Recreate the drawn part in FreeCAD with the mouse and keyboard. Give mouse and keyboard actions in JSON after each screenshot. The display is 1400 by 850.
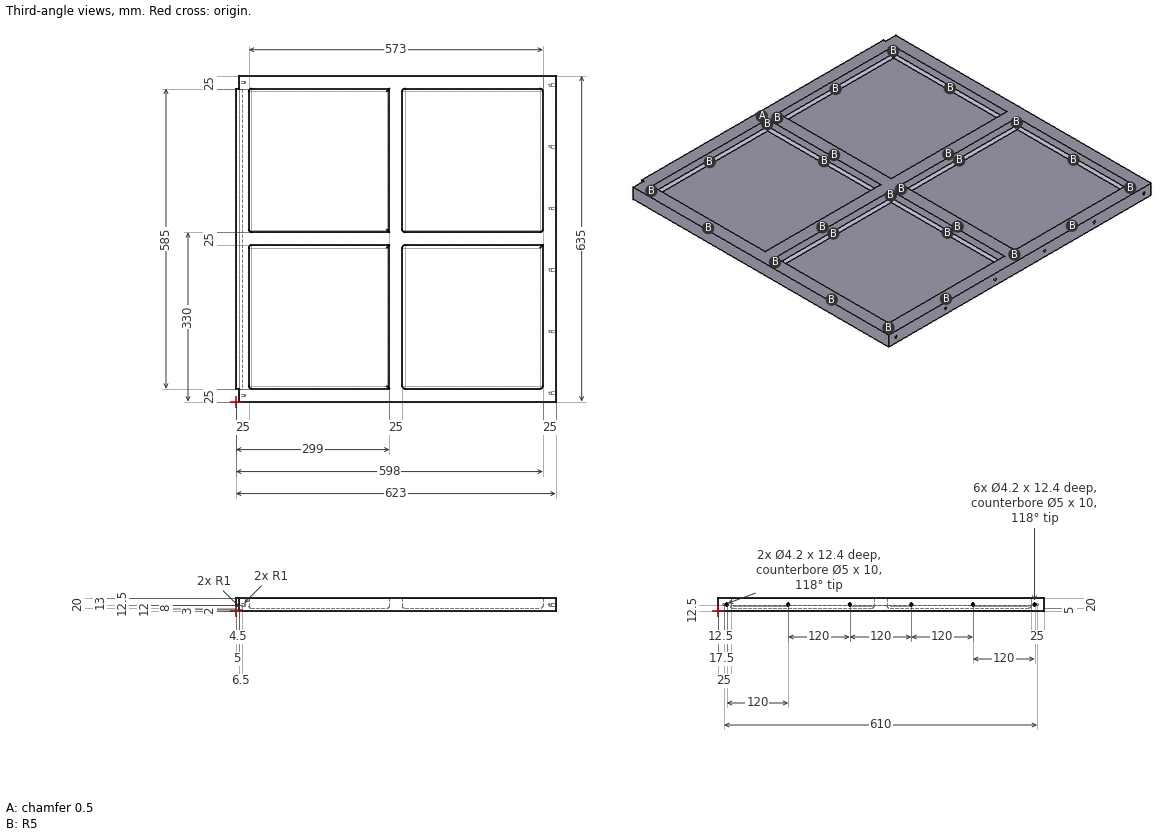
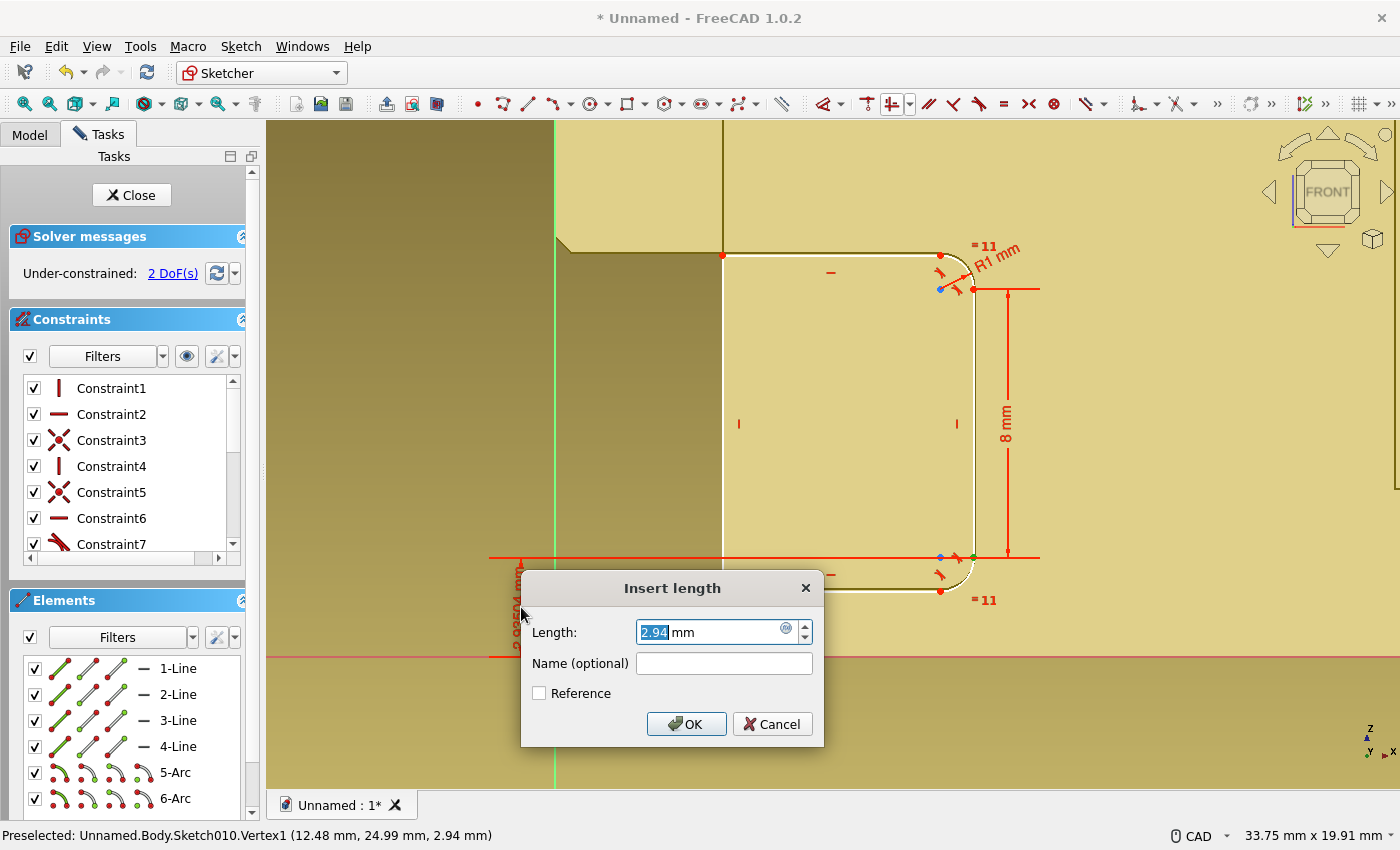
{"action": "type", "text": "3"}
{"action": "key", "text": "Return"}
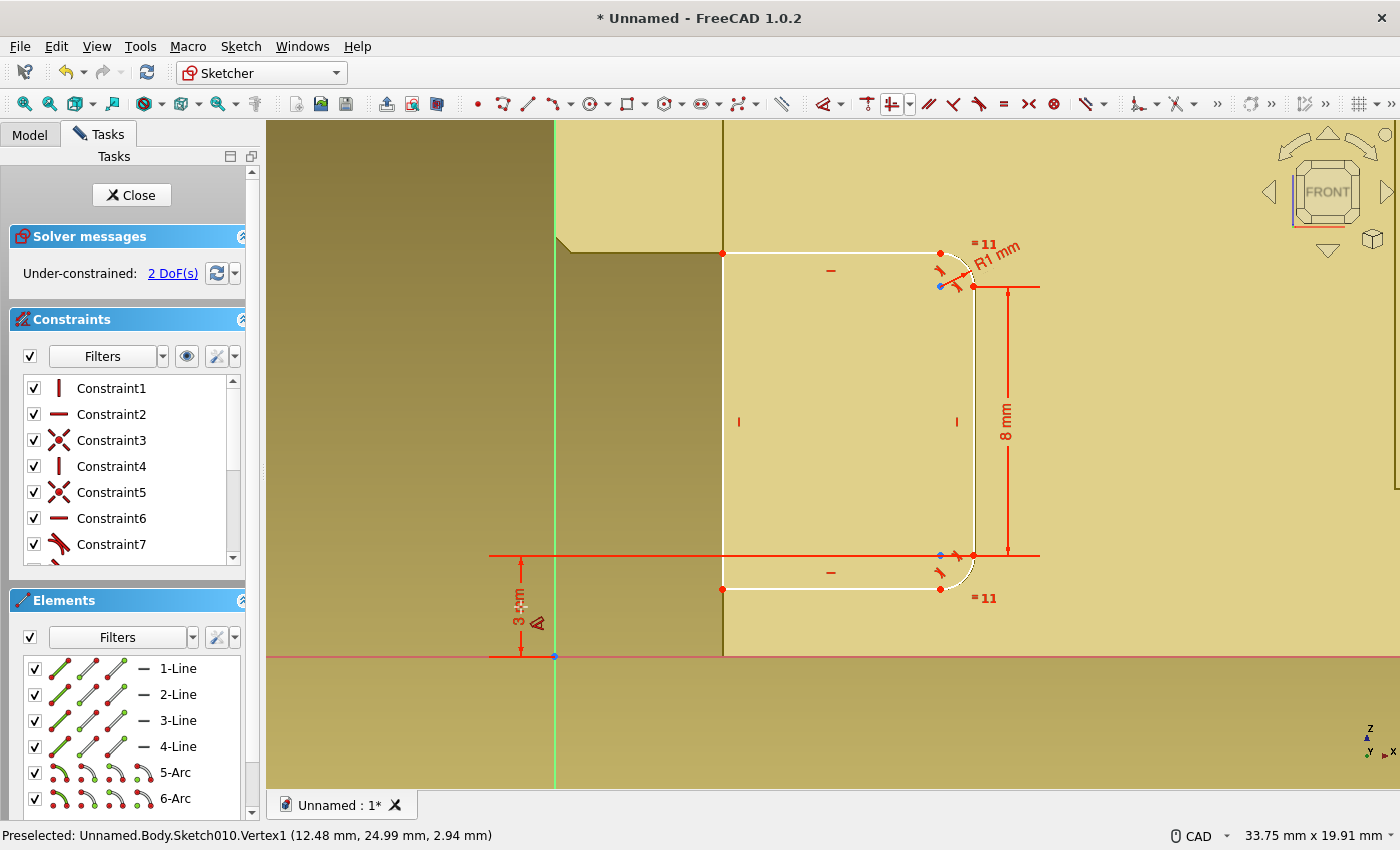
{"action": "left_click", "coordinate": [723, 253]}
{"action": "left_click", "coordinate": [639, 691]}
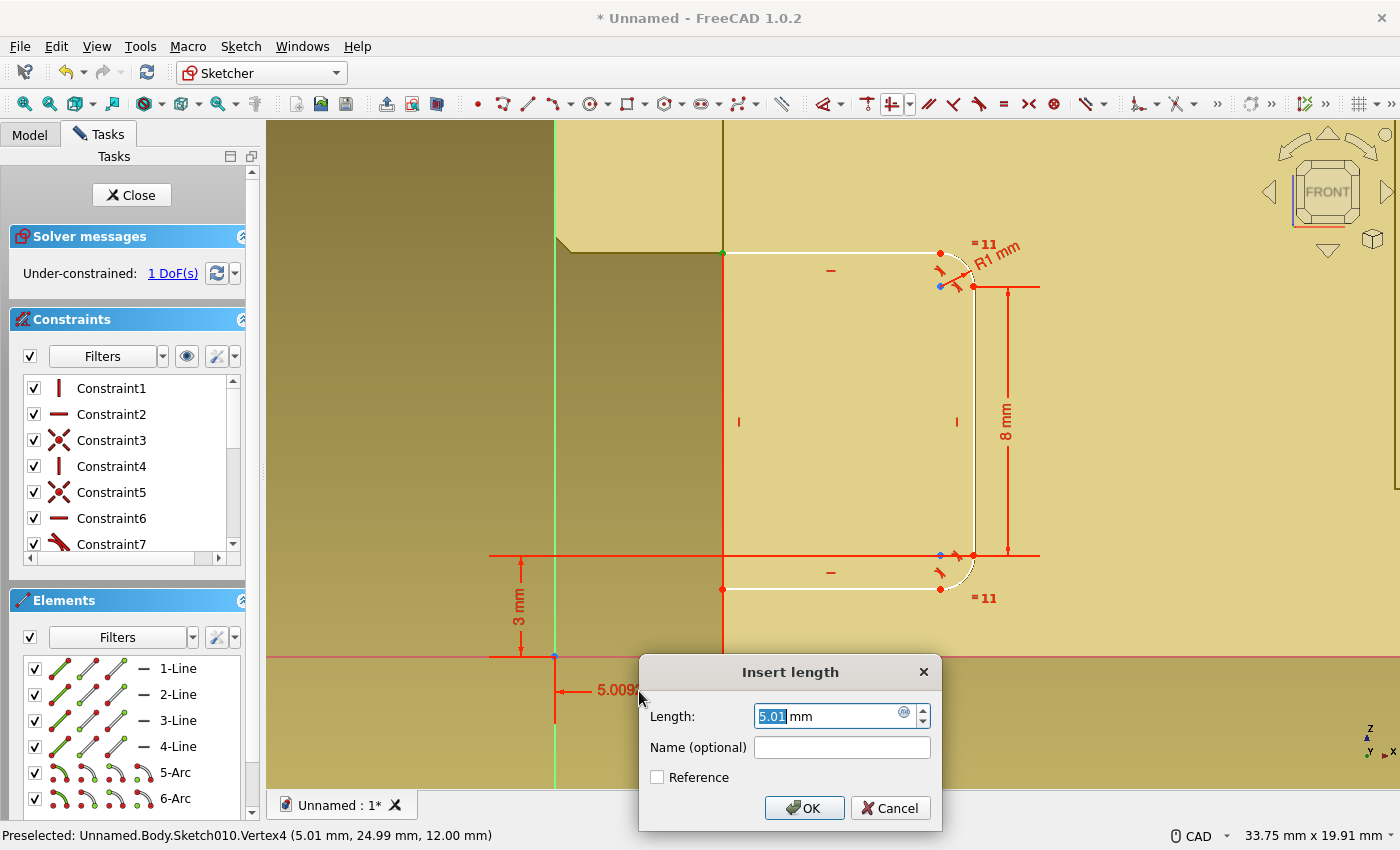
{"action": "type", "text": "5"}
{"action": "key", "text": "Return"}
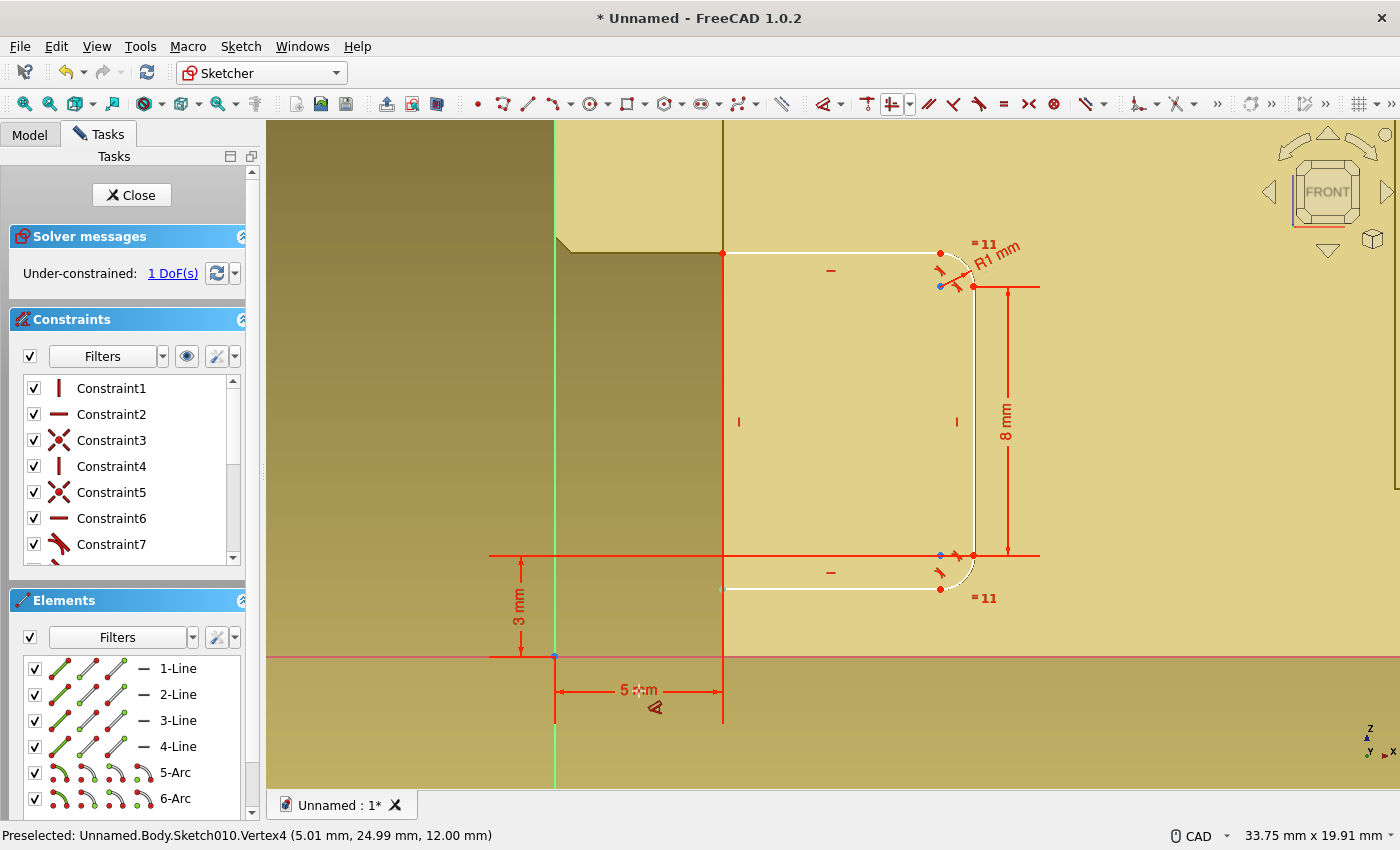
{"action": "left_click", "coordinate": [875, 253]}
{"action": "left_click", "coordinate": [831, 219]}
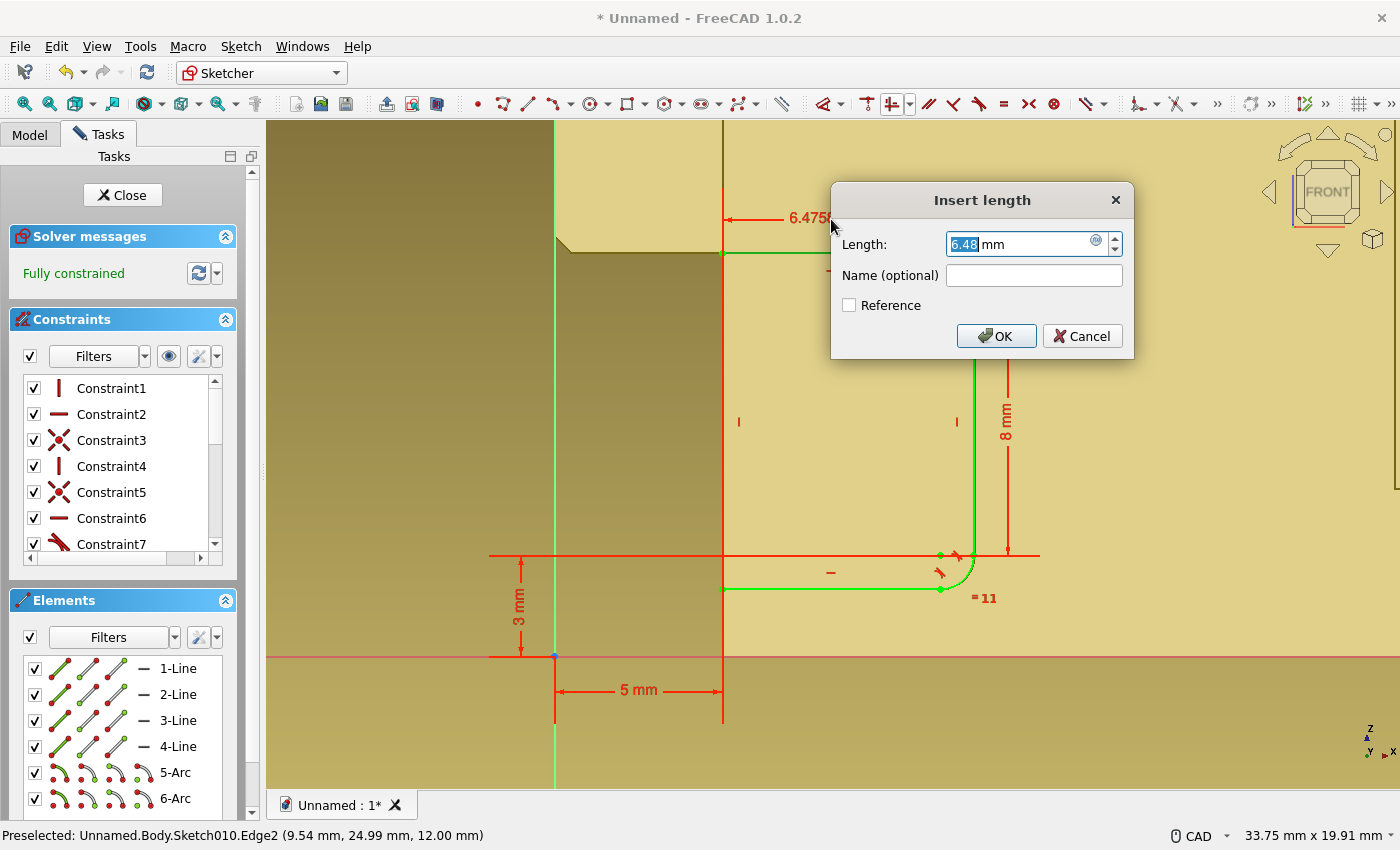
{"action": "type", "text": "6.5"}
{"action": "key", "text": "Return"}
{"action": "key", "text": "Escape"}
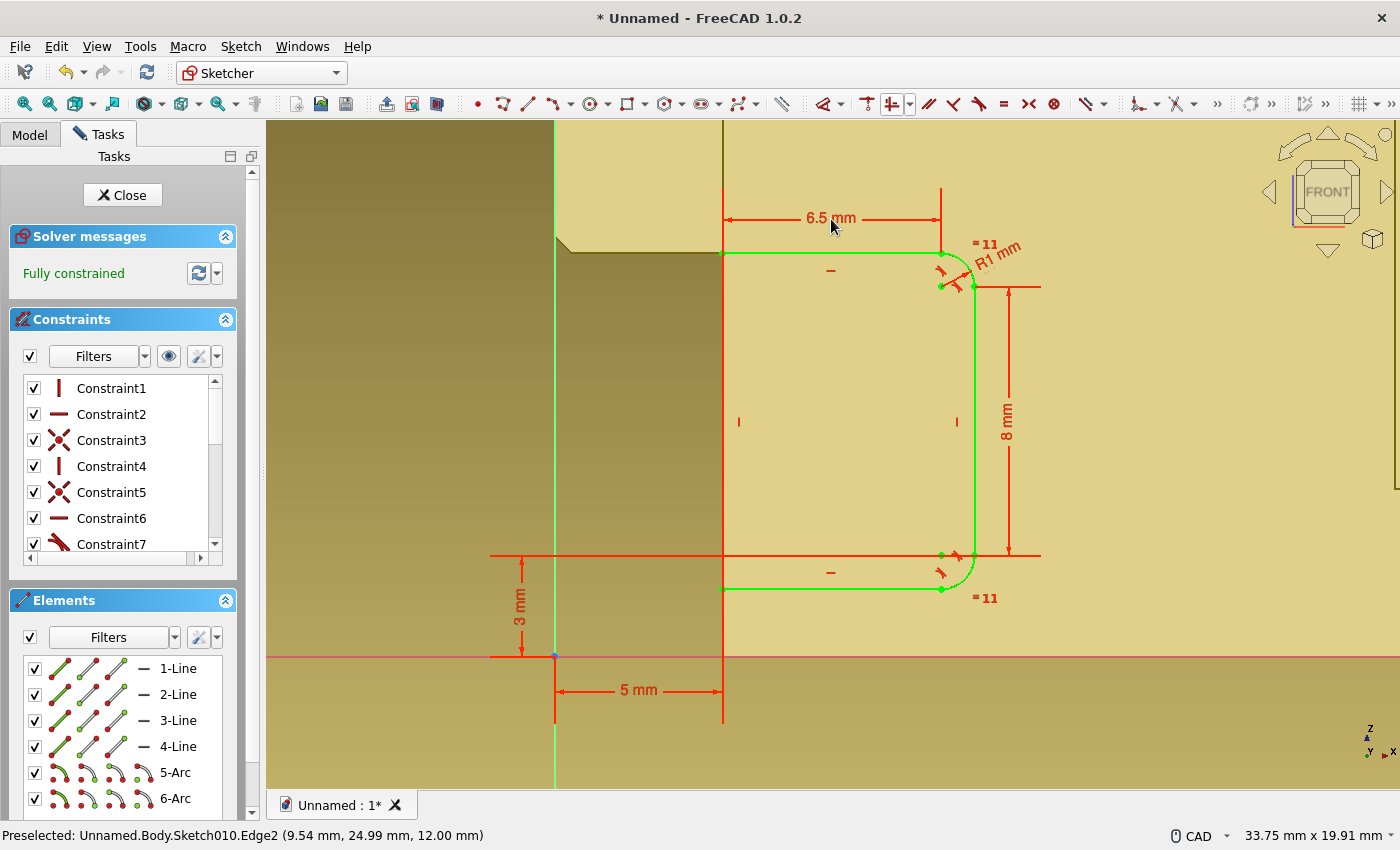
{"action": "left_click", "coordinate": [123, 195]}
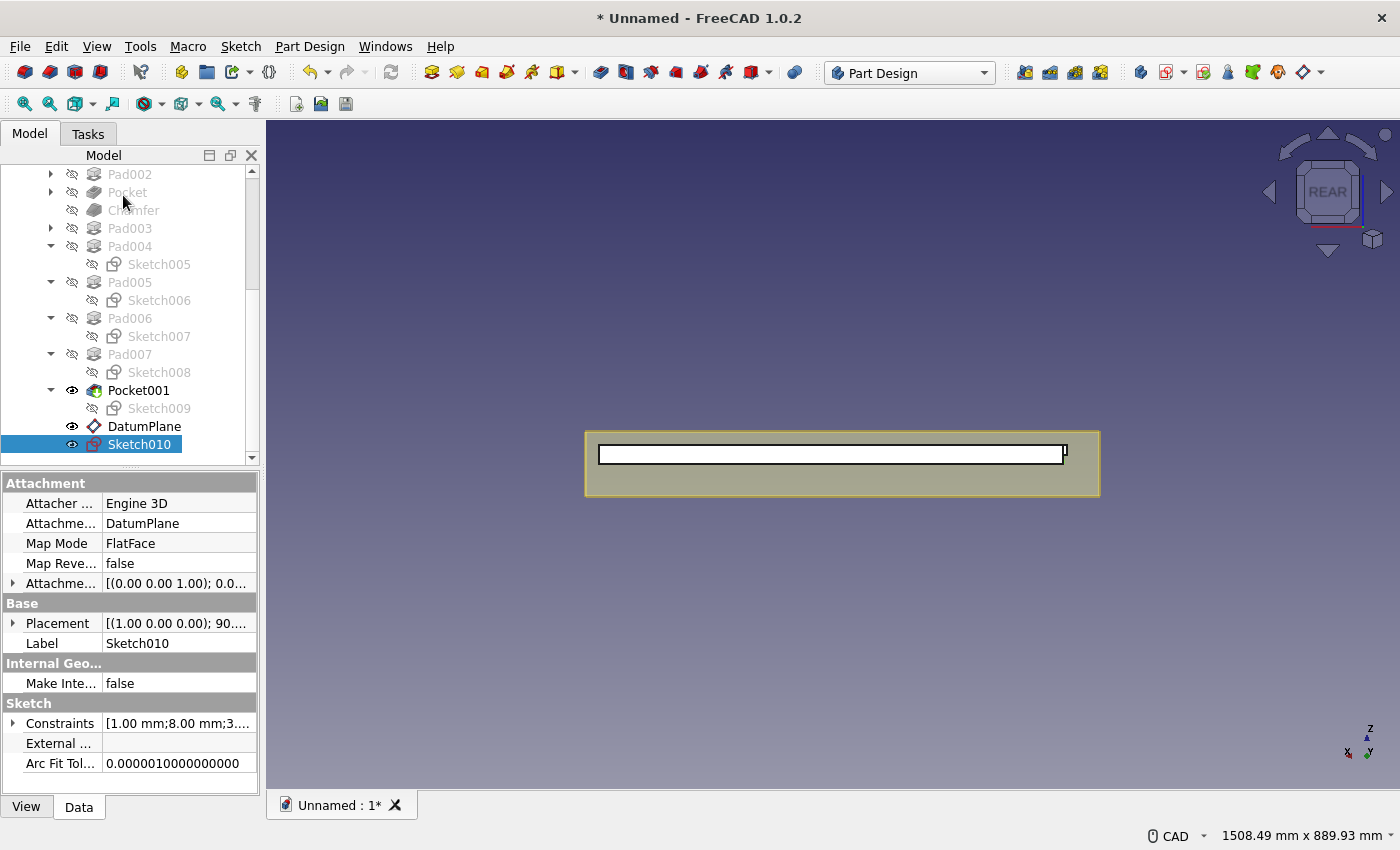
{"action": "left_click", "coordinate": [432, 72]}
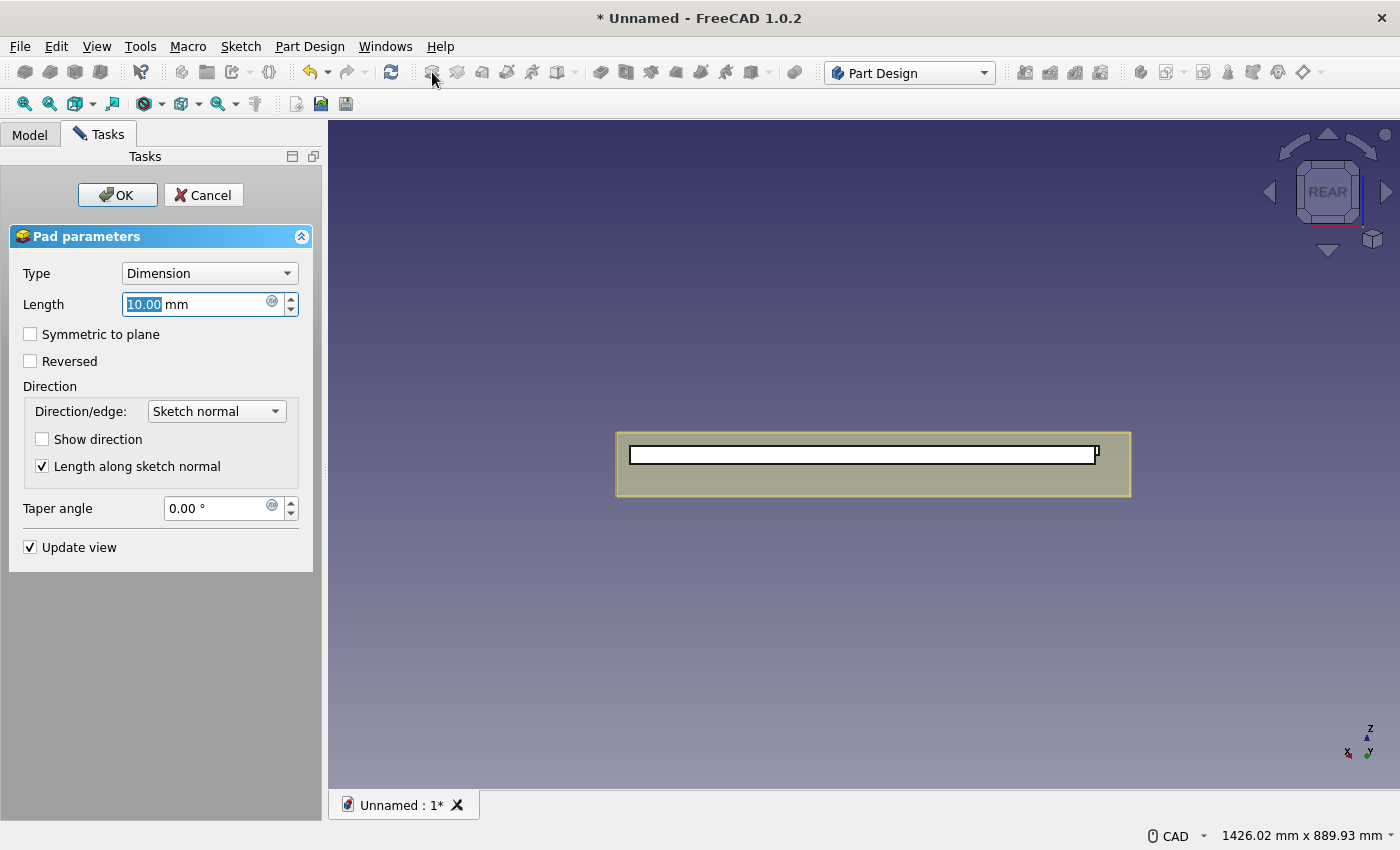
{"action": "type", "text": "25"}
{"action": "key", "text": "Tab"}